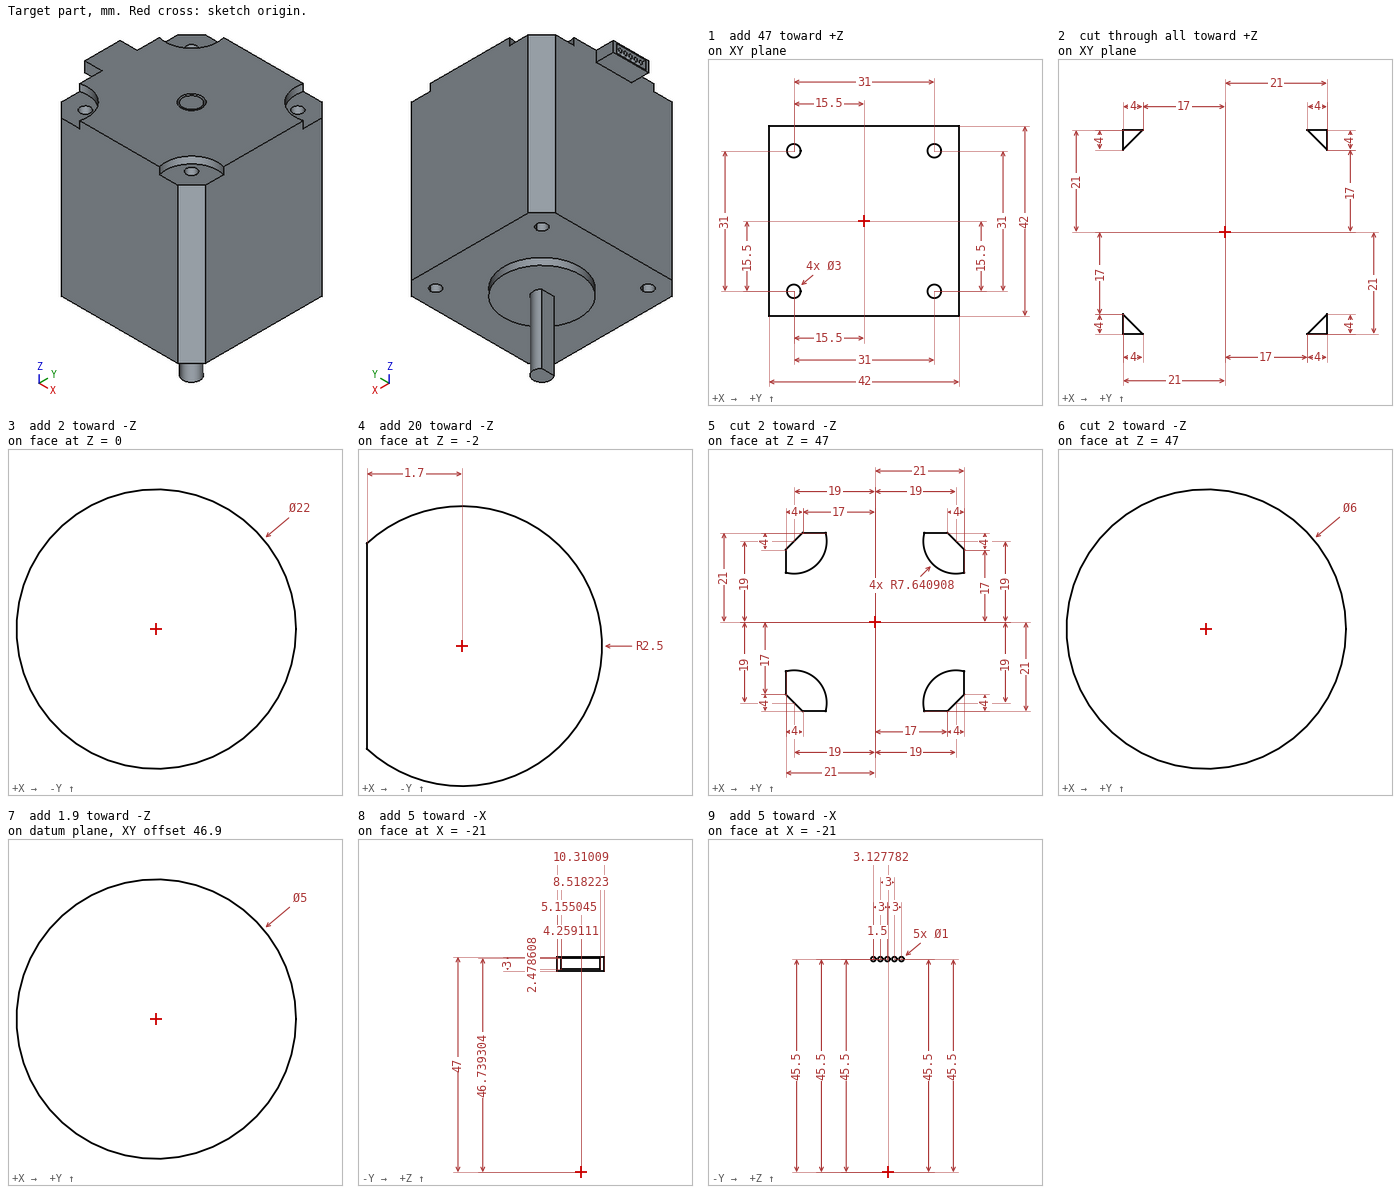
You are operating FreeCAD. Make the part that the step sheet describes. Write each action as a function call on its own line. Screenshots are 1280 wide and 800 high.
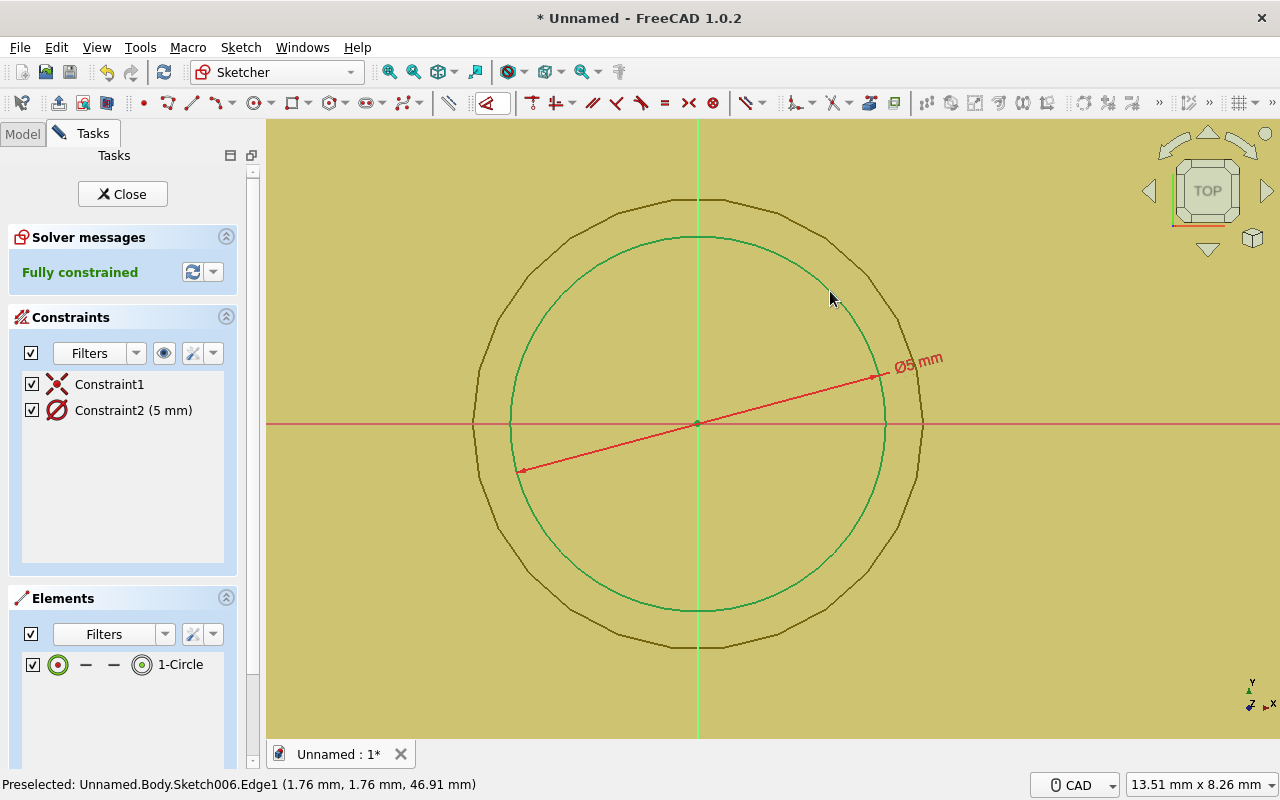
click(123, 194)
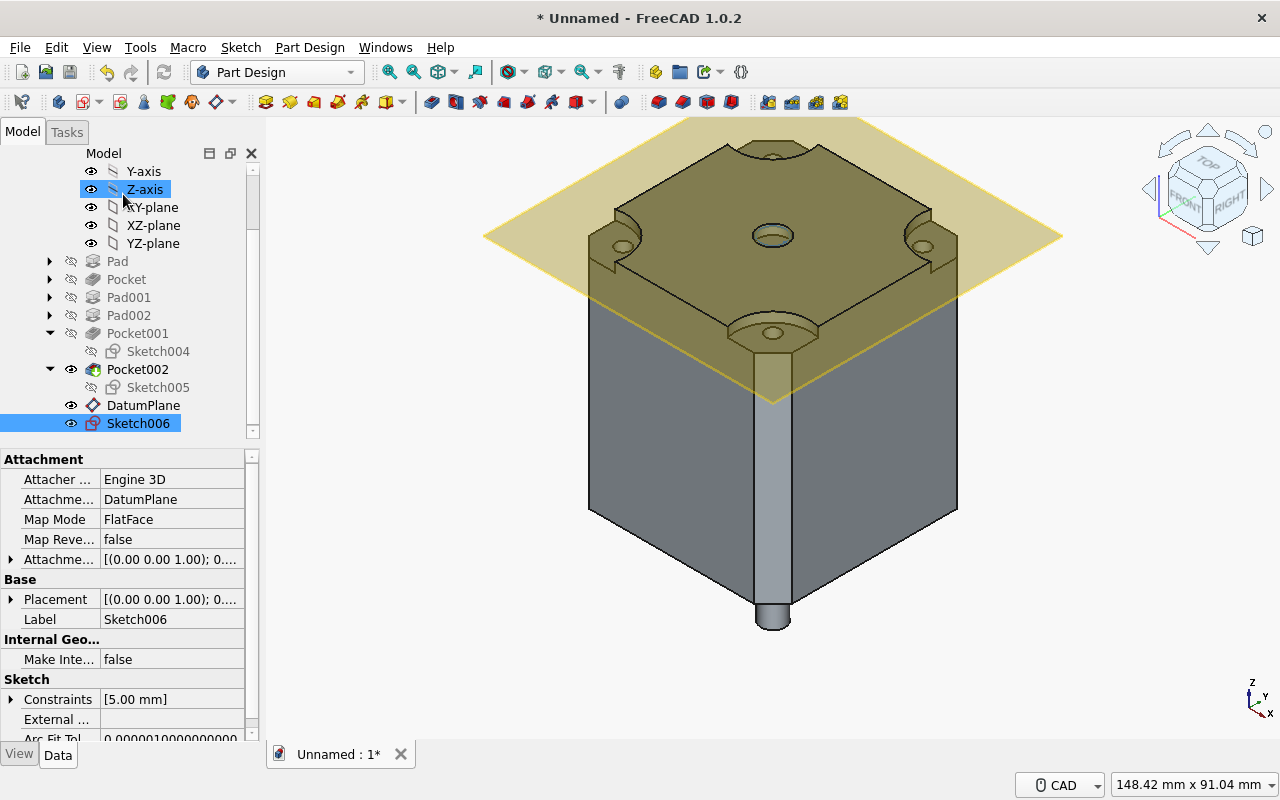
click(266, 102)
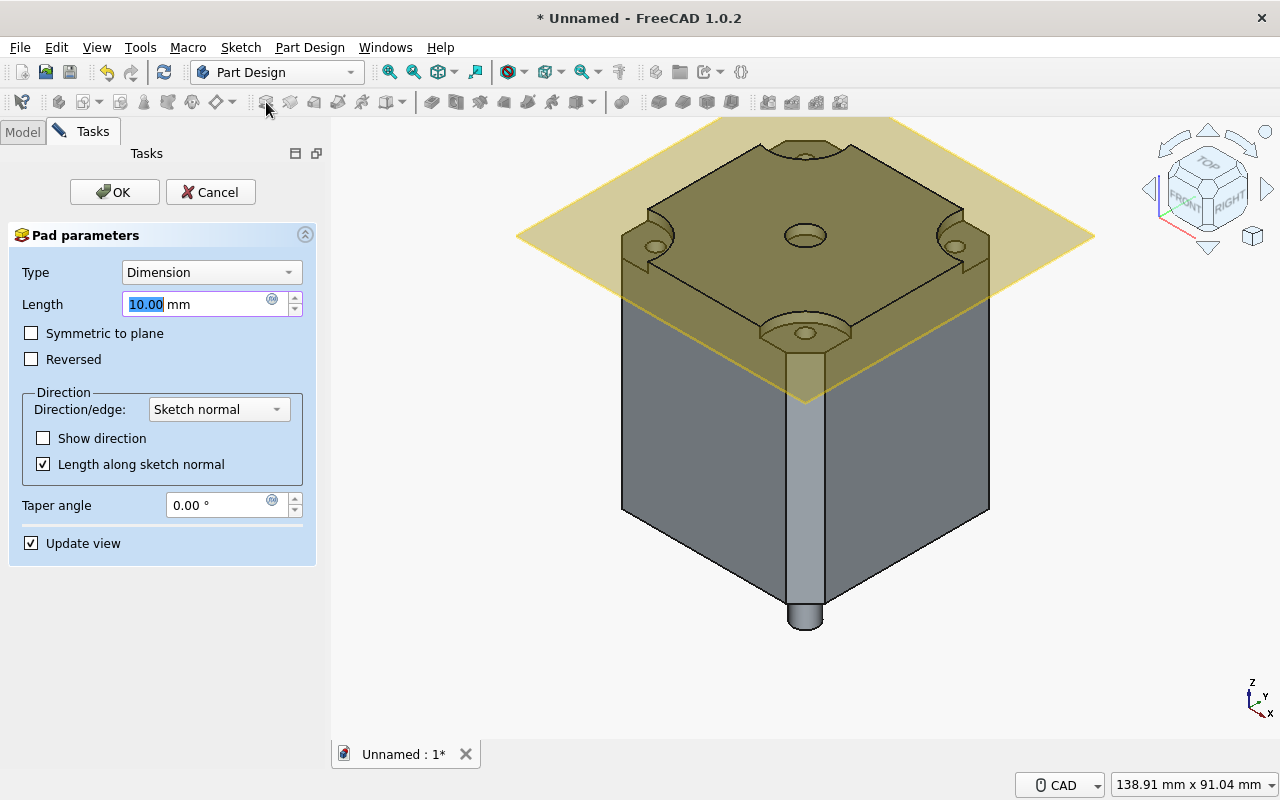
text(1.9)
key(Tab)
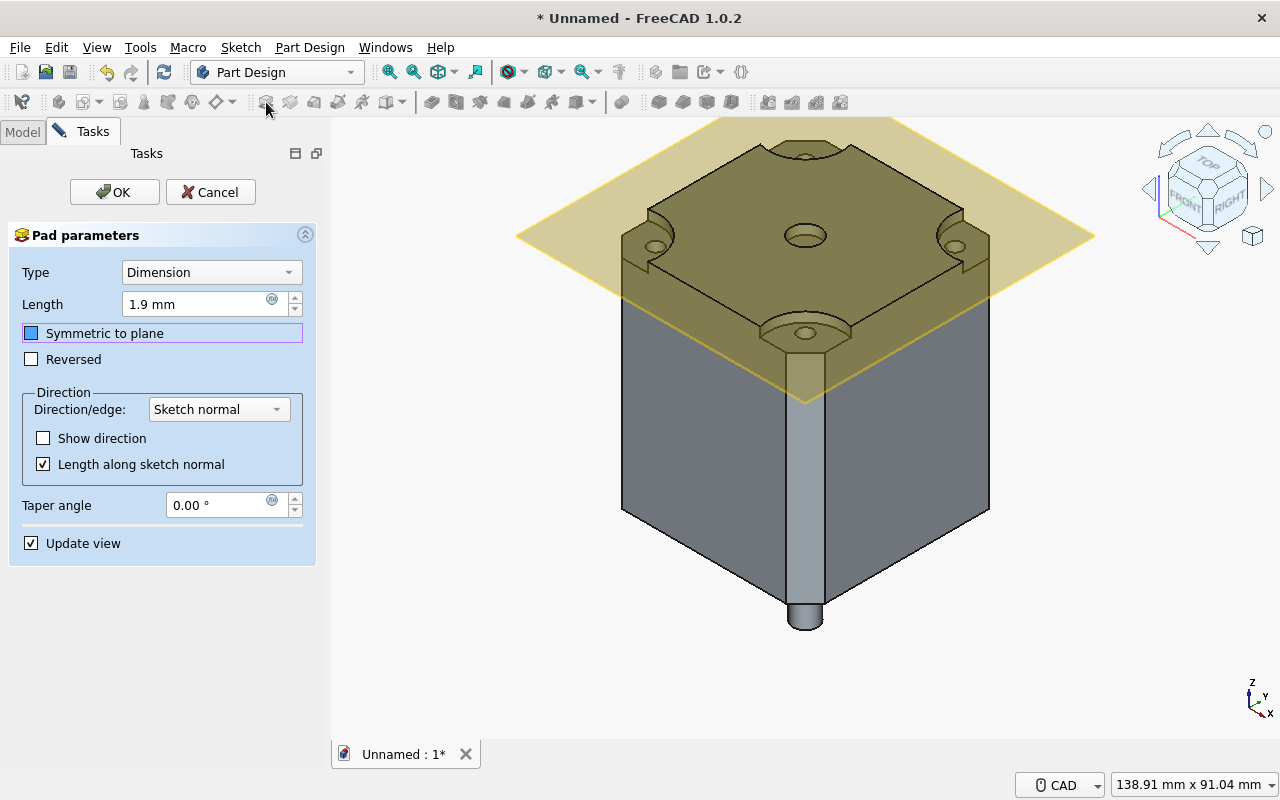
click(30, 359)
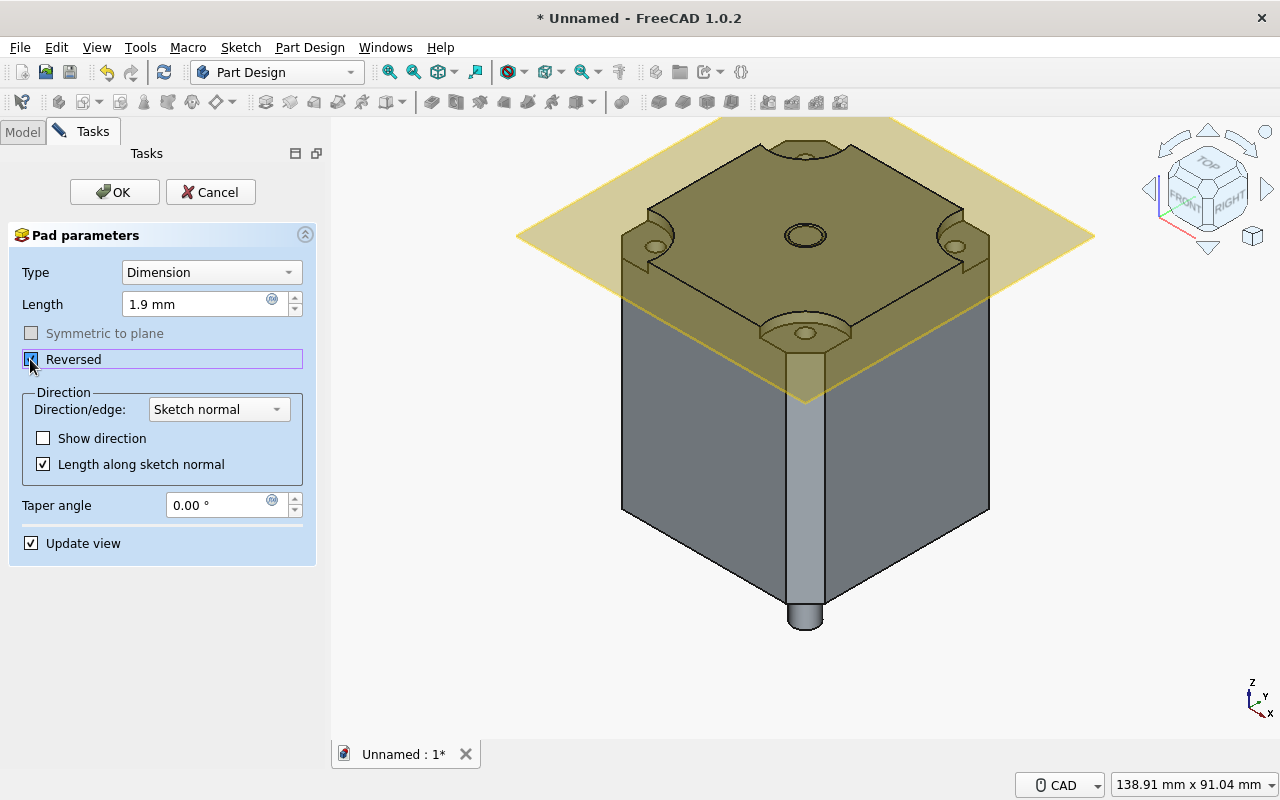
click(115, 192)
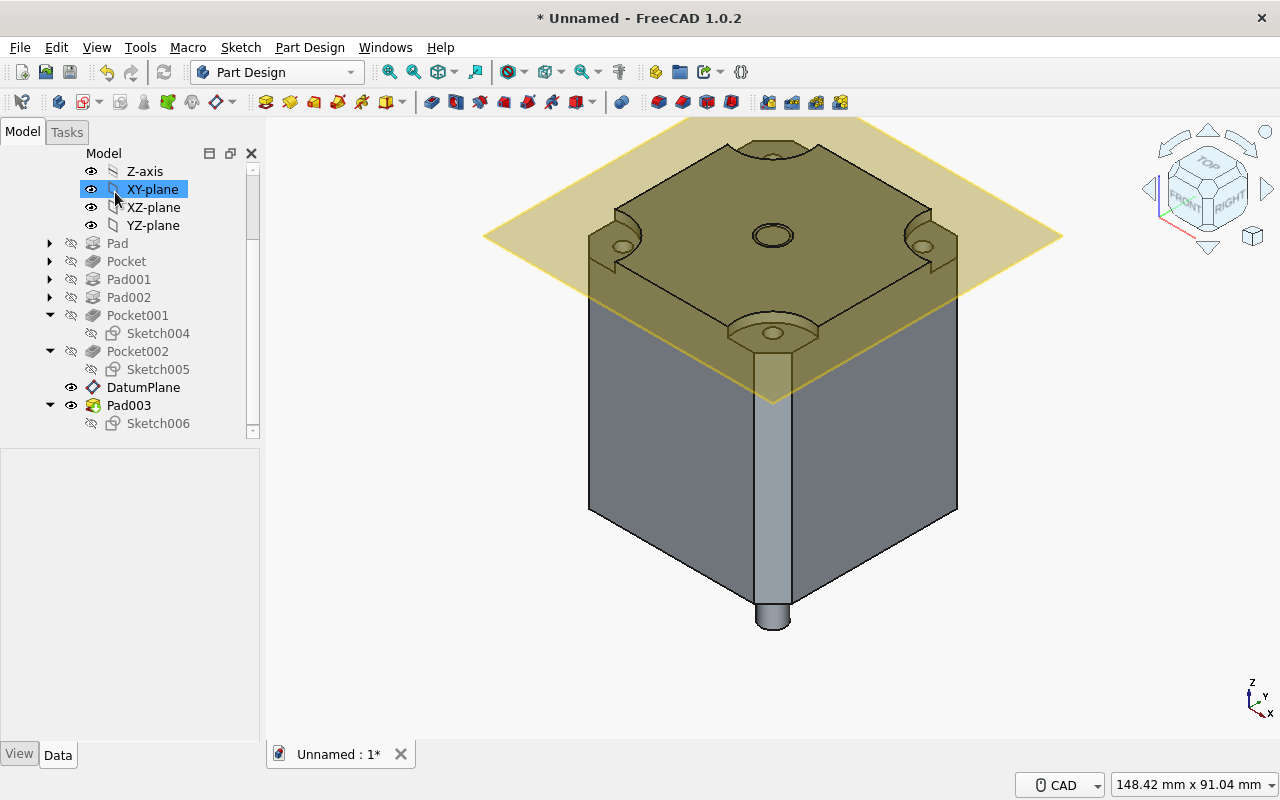
click(116, 387)
key(space)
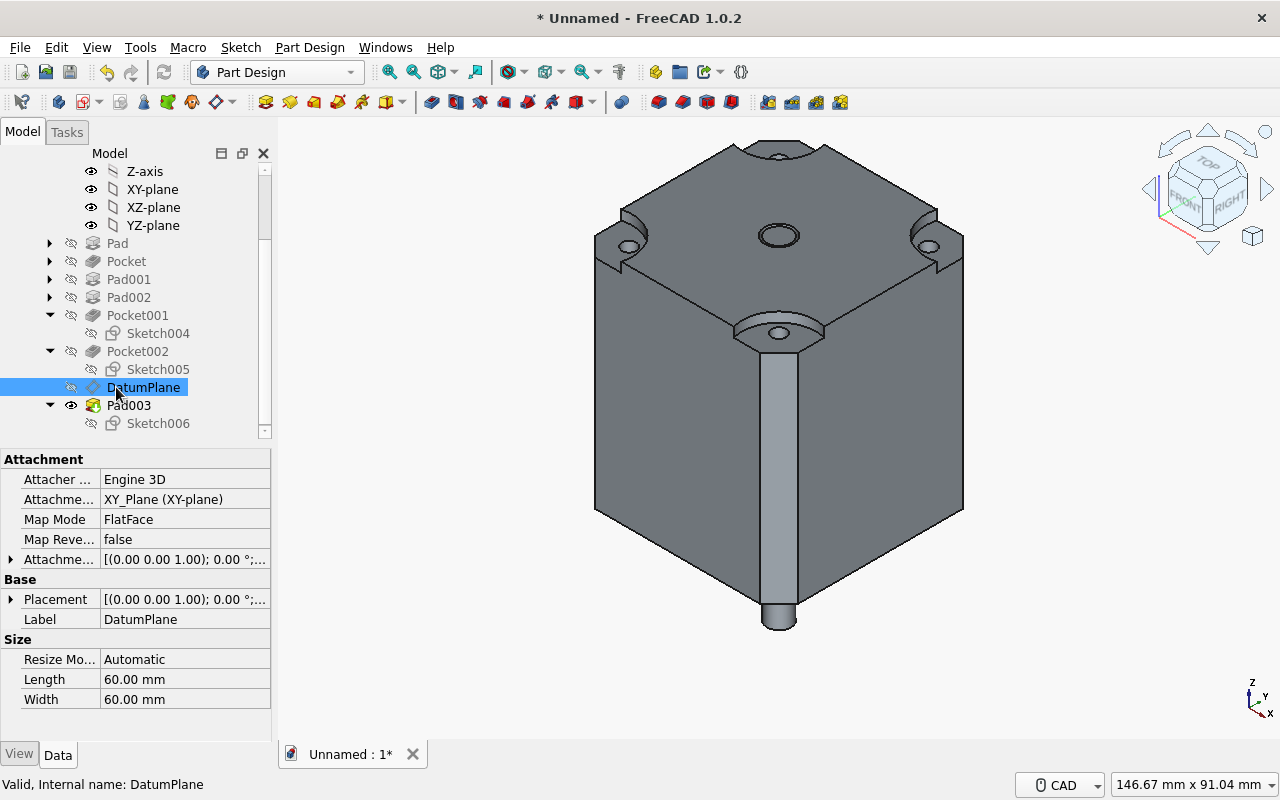
key(6)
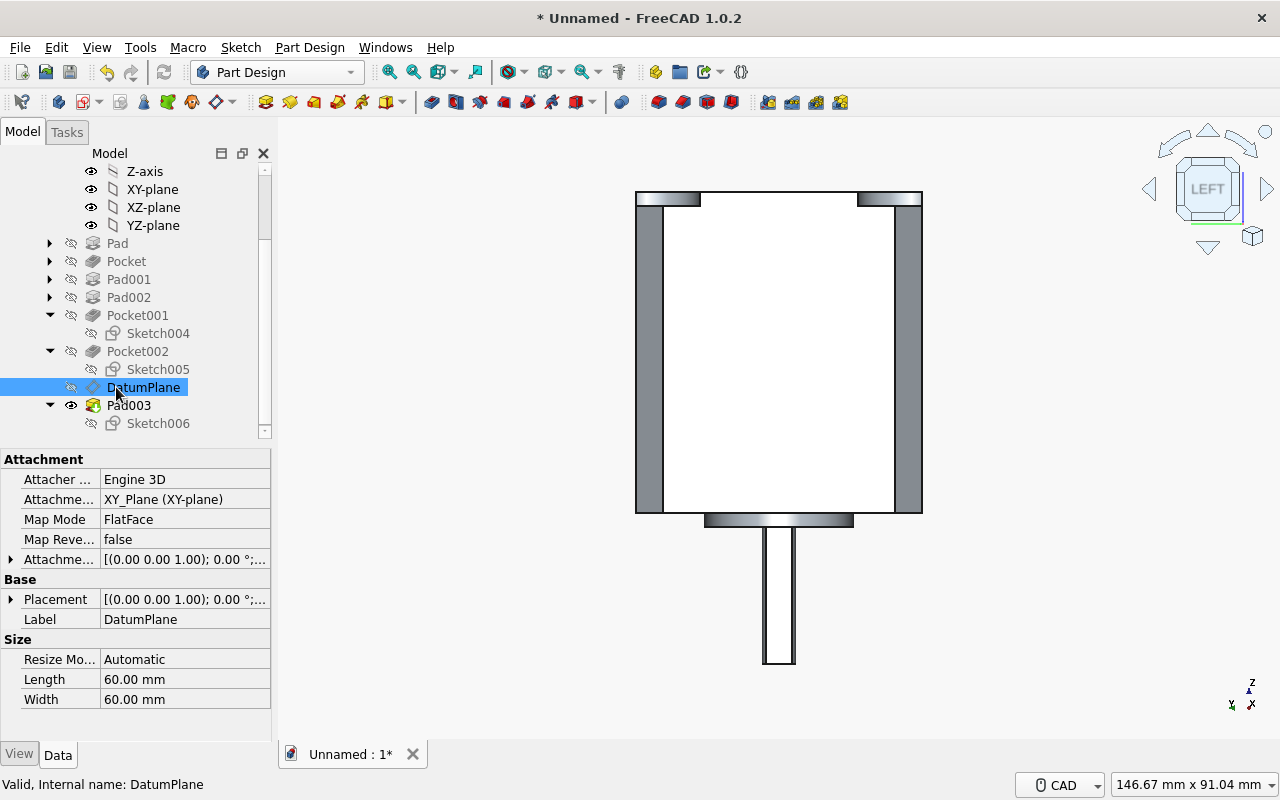
click(779, 352)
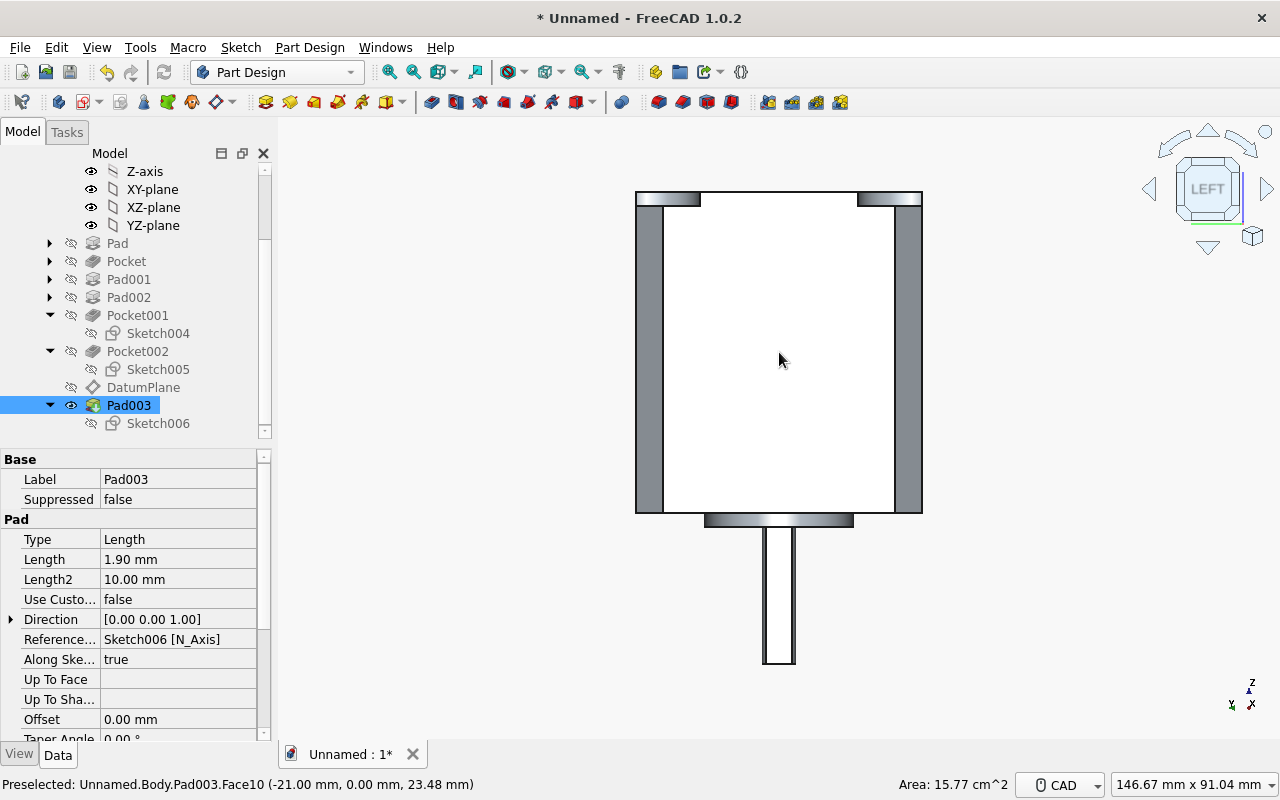
click(84, 102)